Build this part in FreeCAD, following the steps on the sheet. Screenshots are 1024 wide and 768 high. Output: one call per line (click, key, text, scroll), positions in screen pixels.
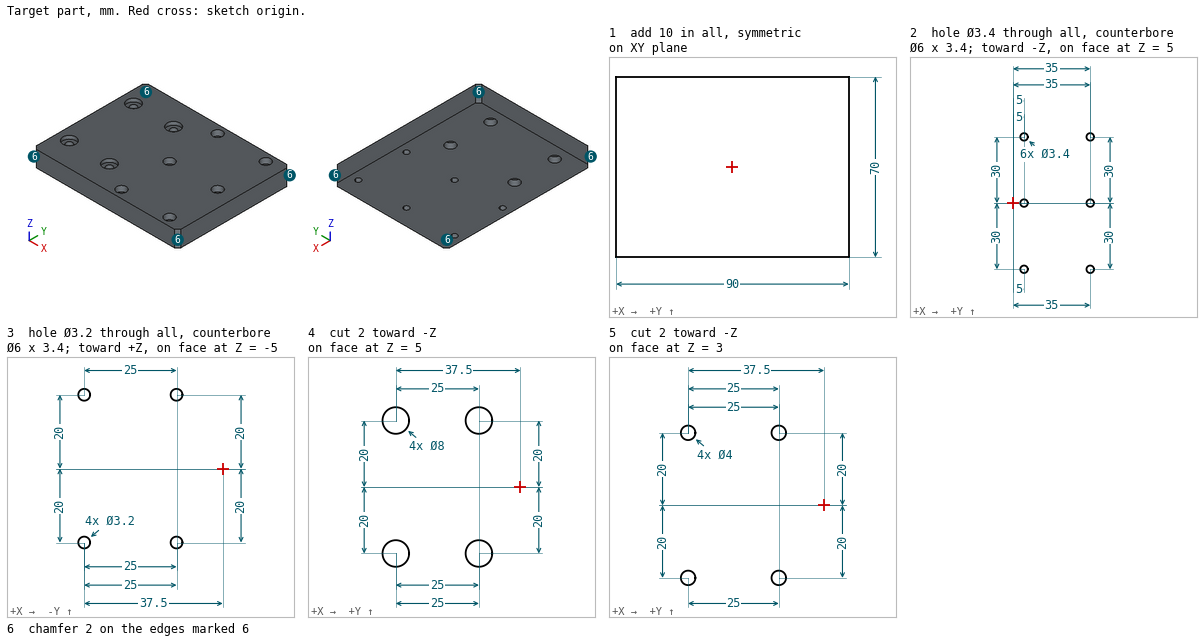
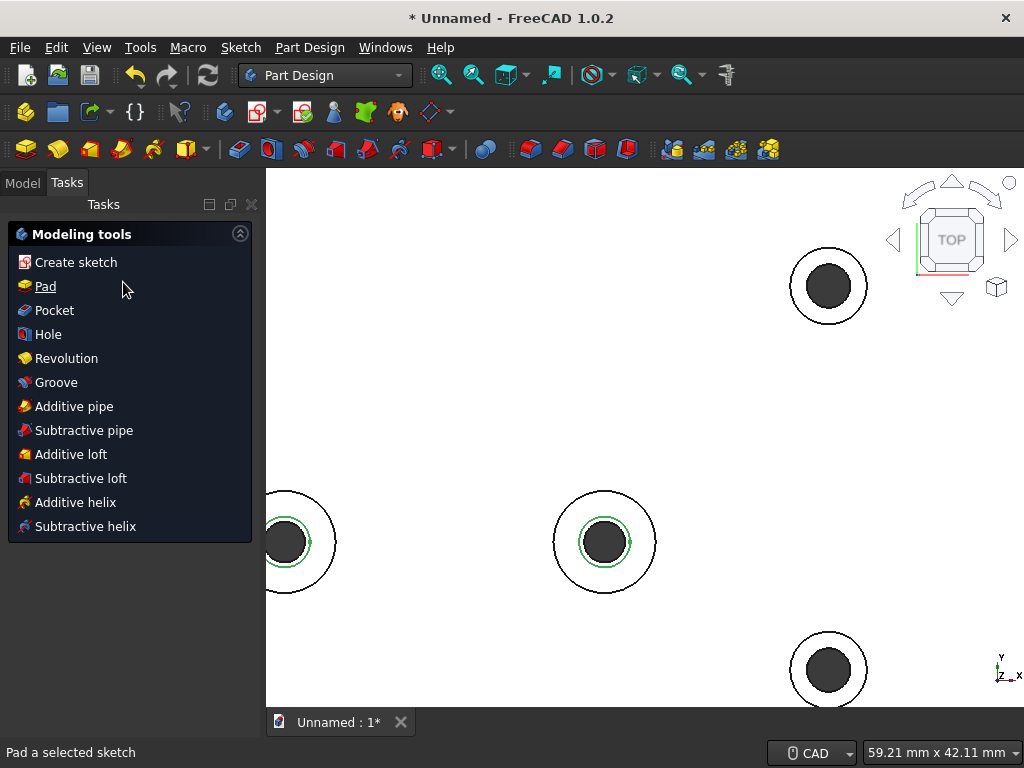
click(240, 150)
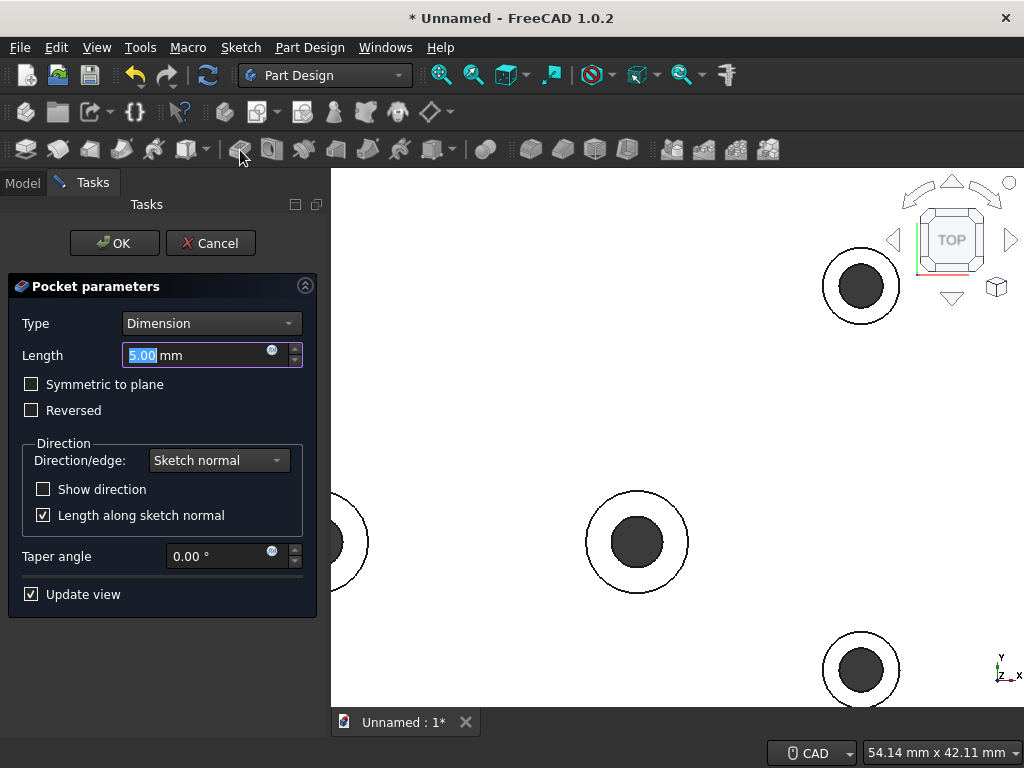
text(2)
key(Tab)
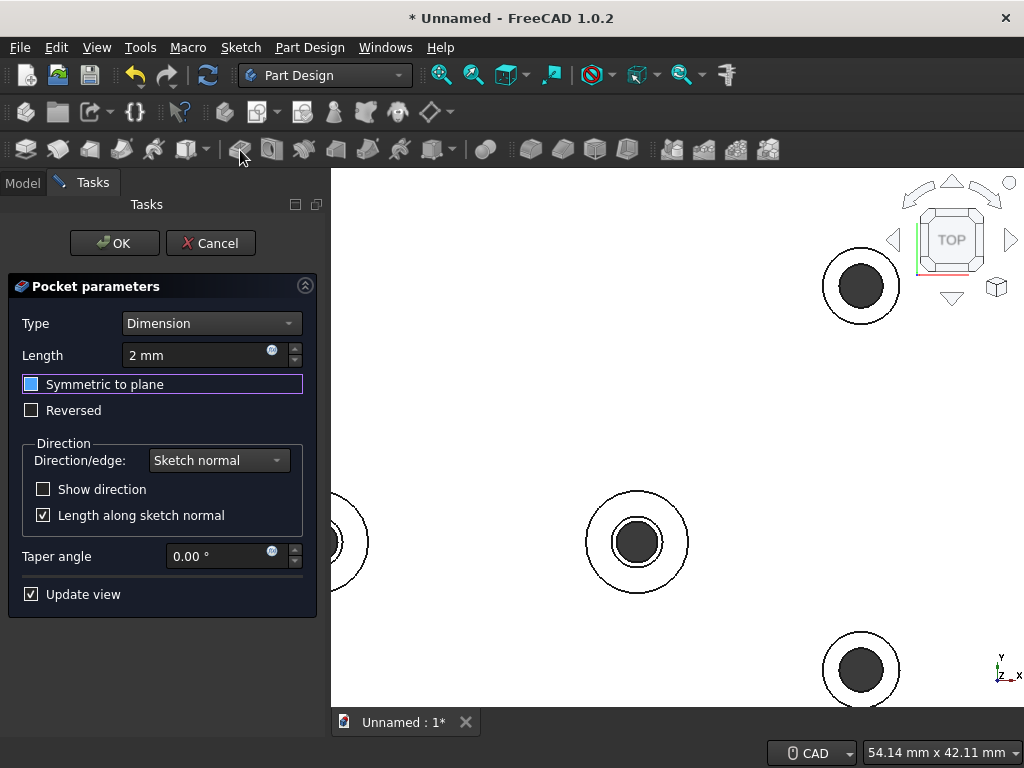
click(115, 243)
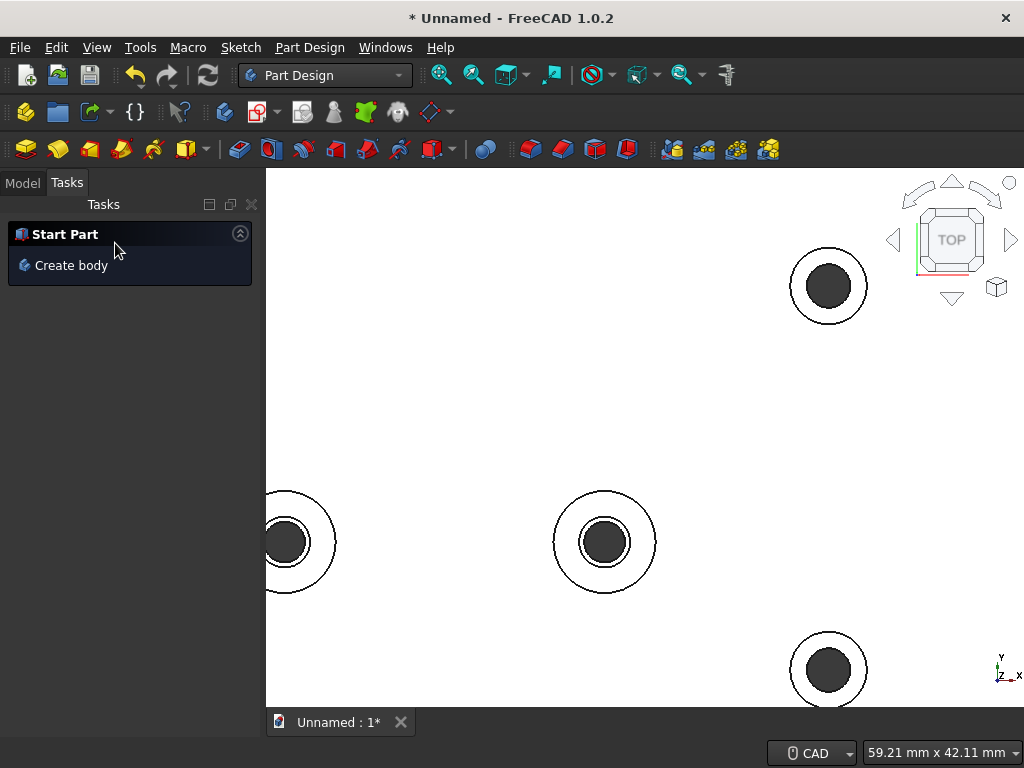
click(442, 76)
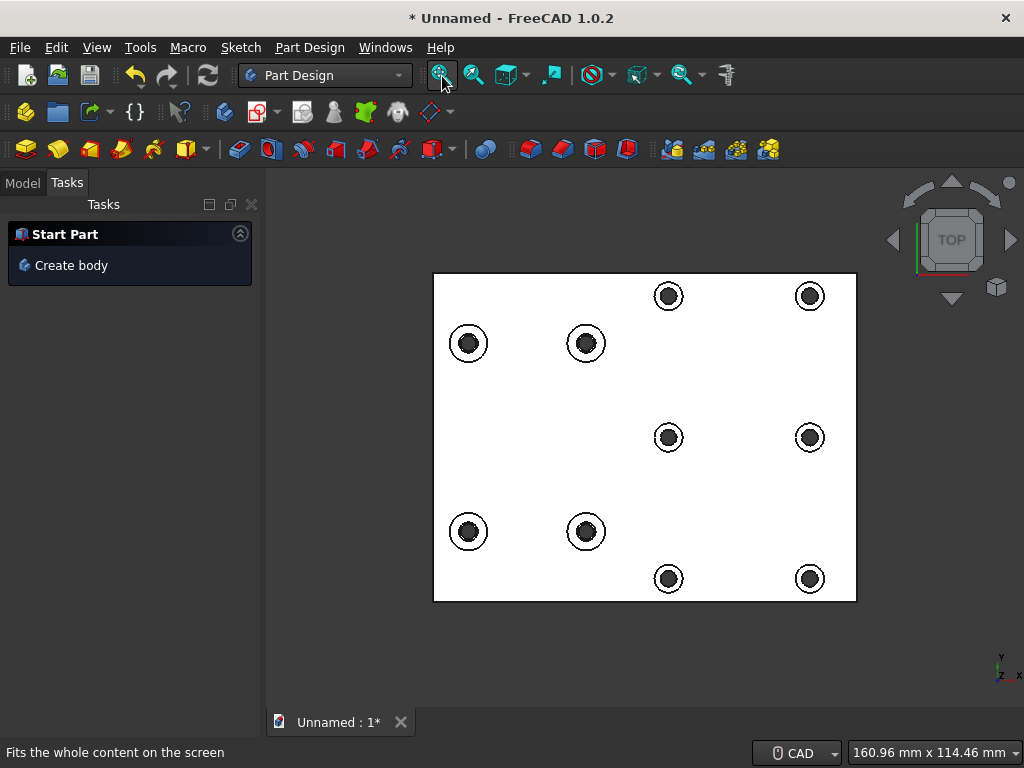
key(0)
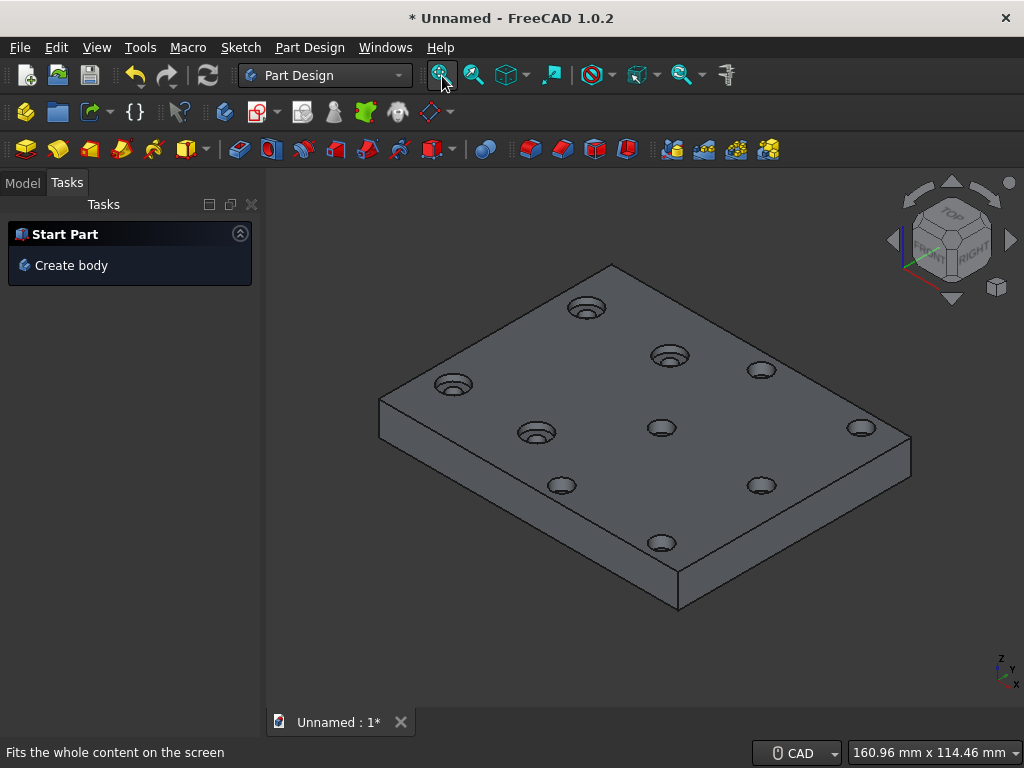
click(678, 590)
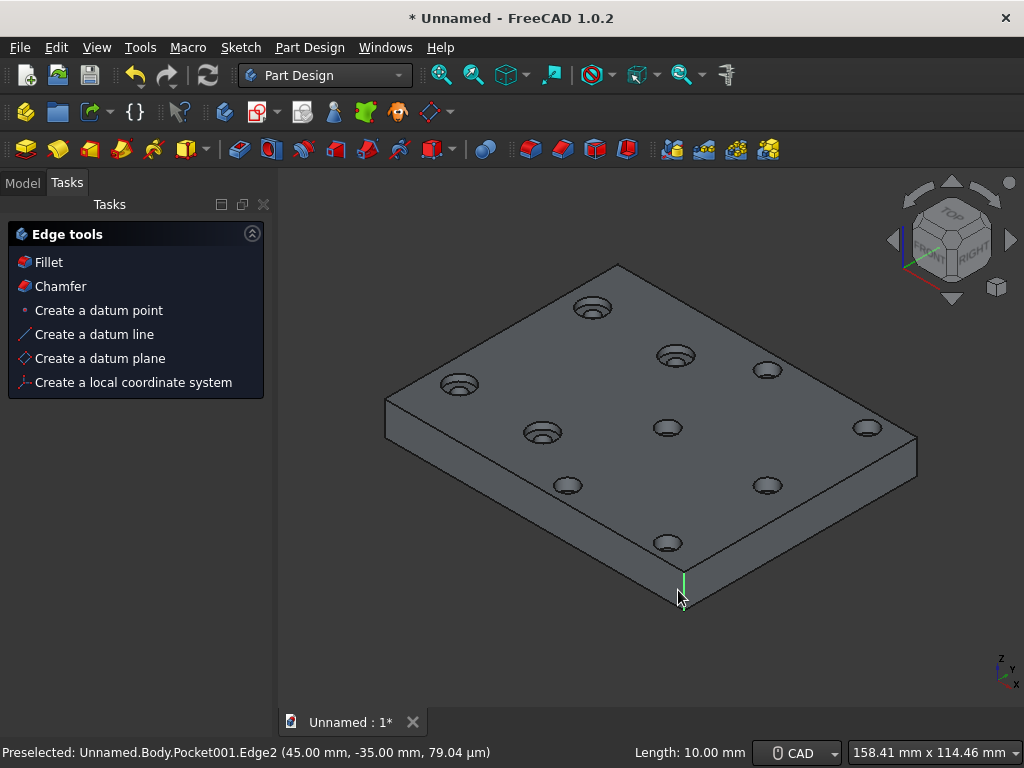
key(2)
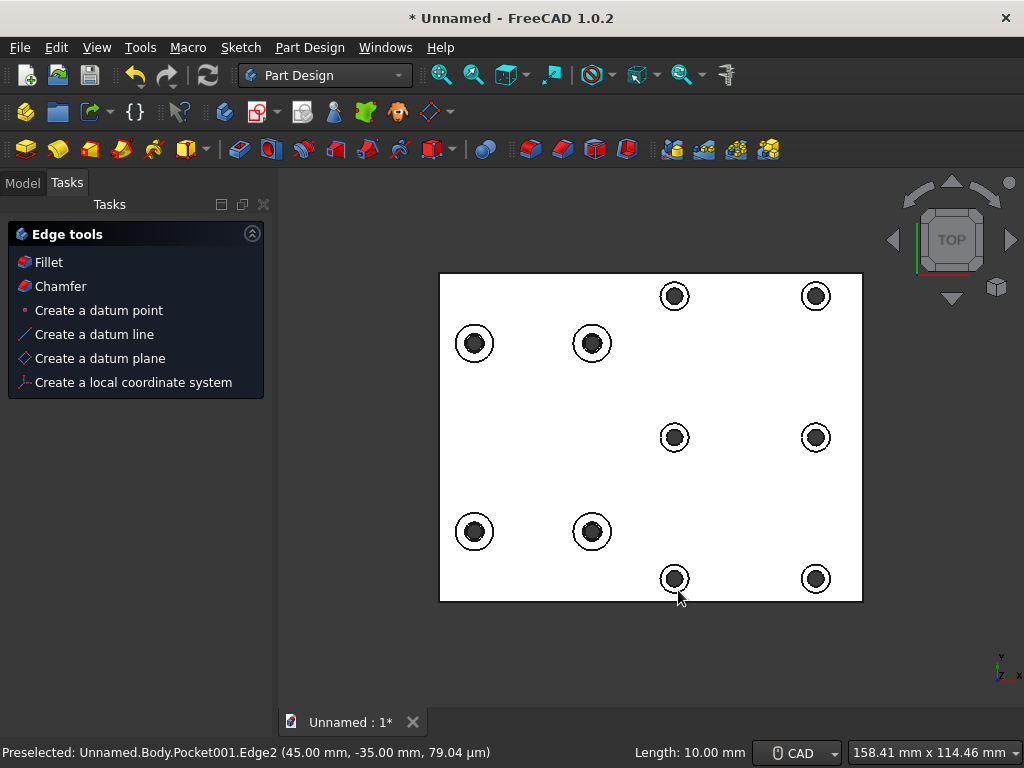
key(1)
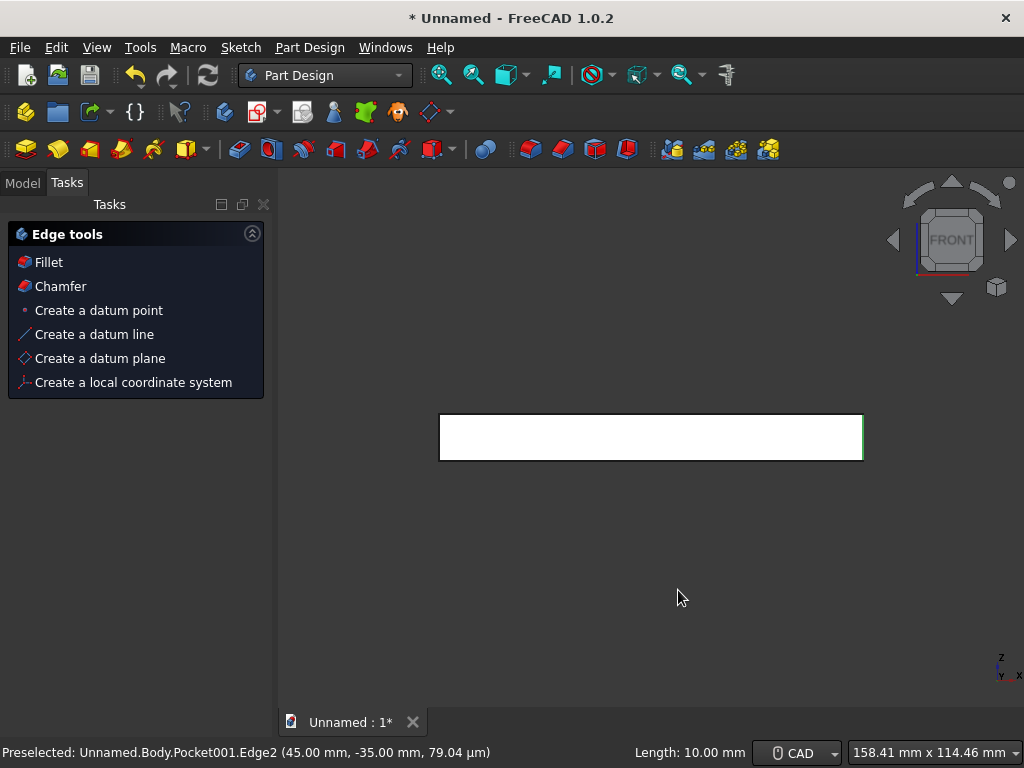
click(439, 436, ctrl)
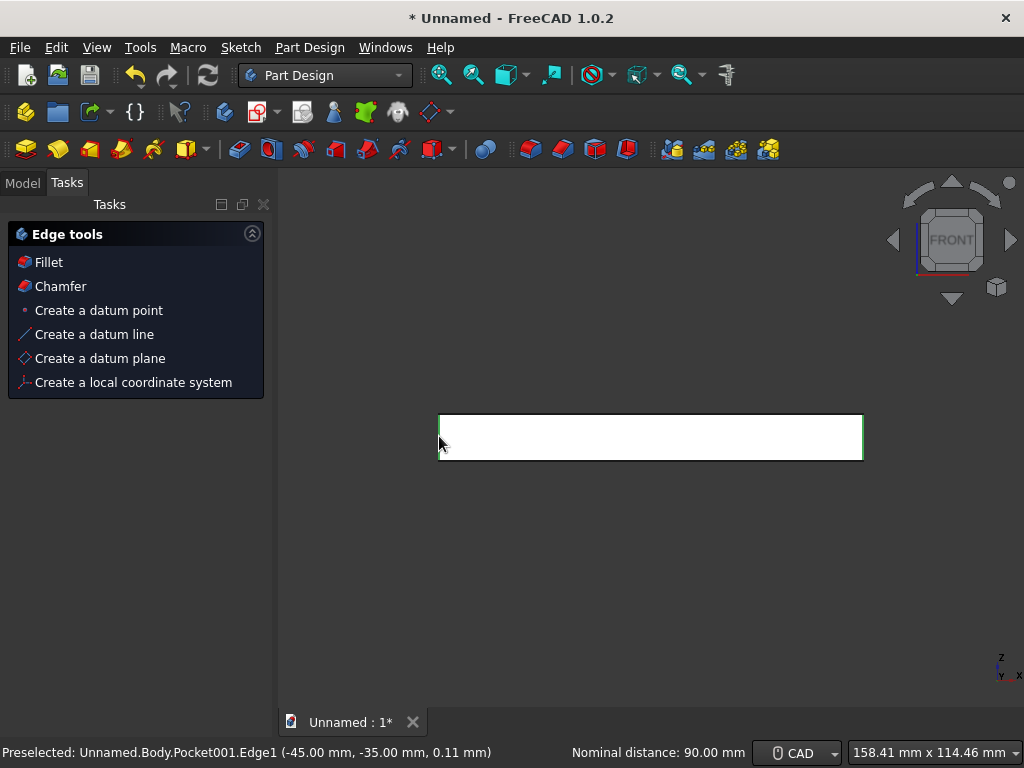
key(3)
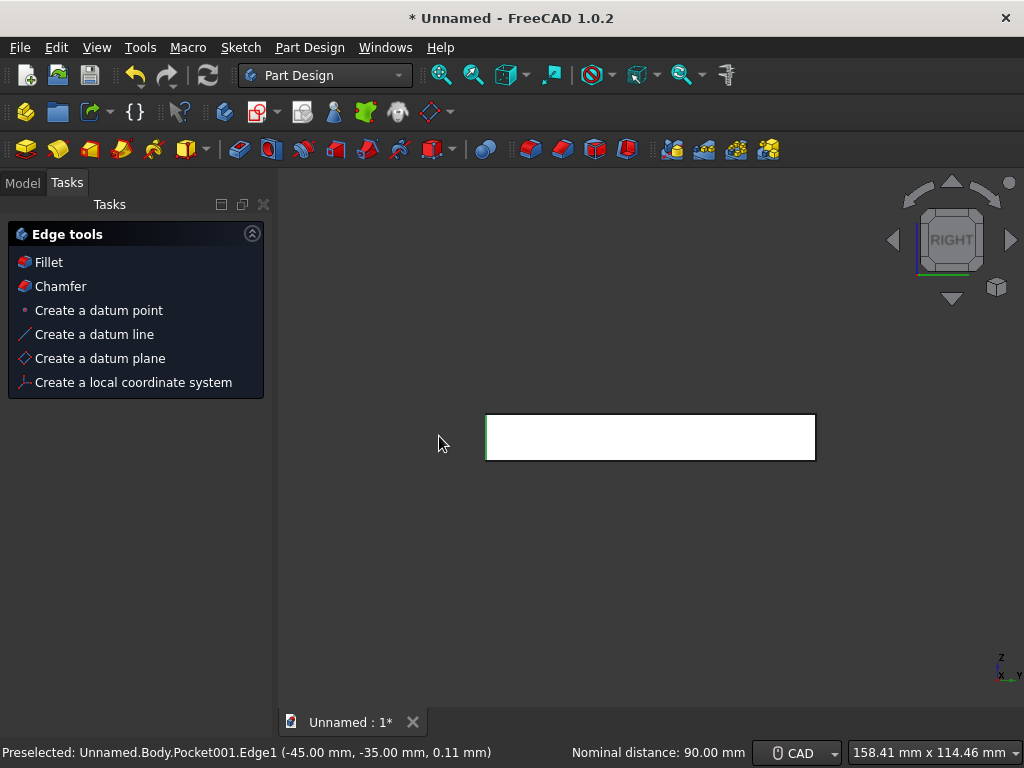
click(442, 76)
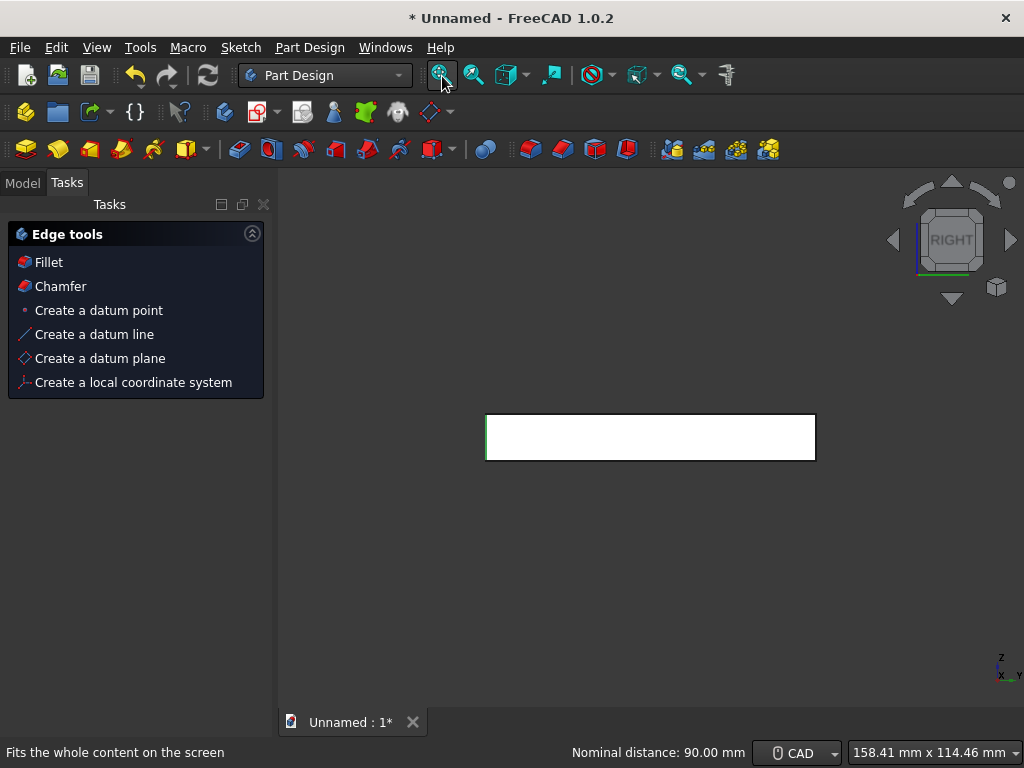
click(816, 436, ctrl)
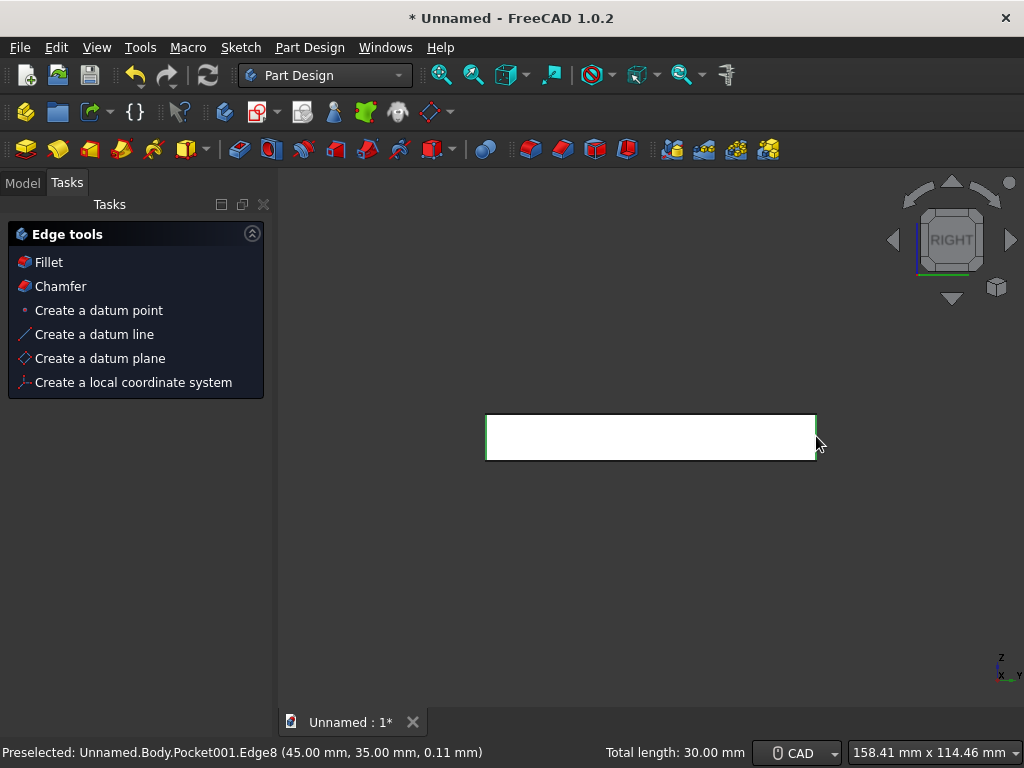
key(5)